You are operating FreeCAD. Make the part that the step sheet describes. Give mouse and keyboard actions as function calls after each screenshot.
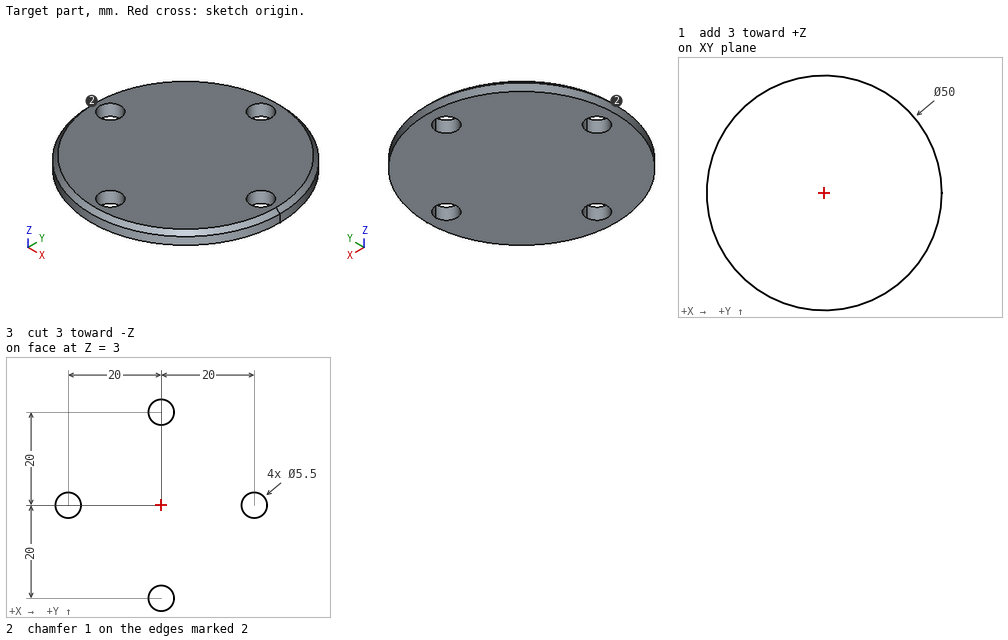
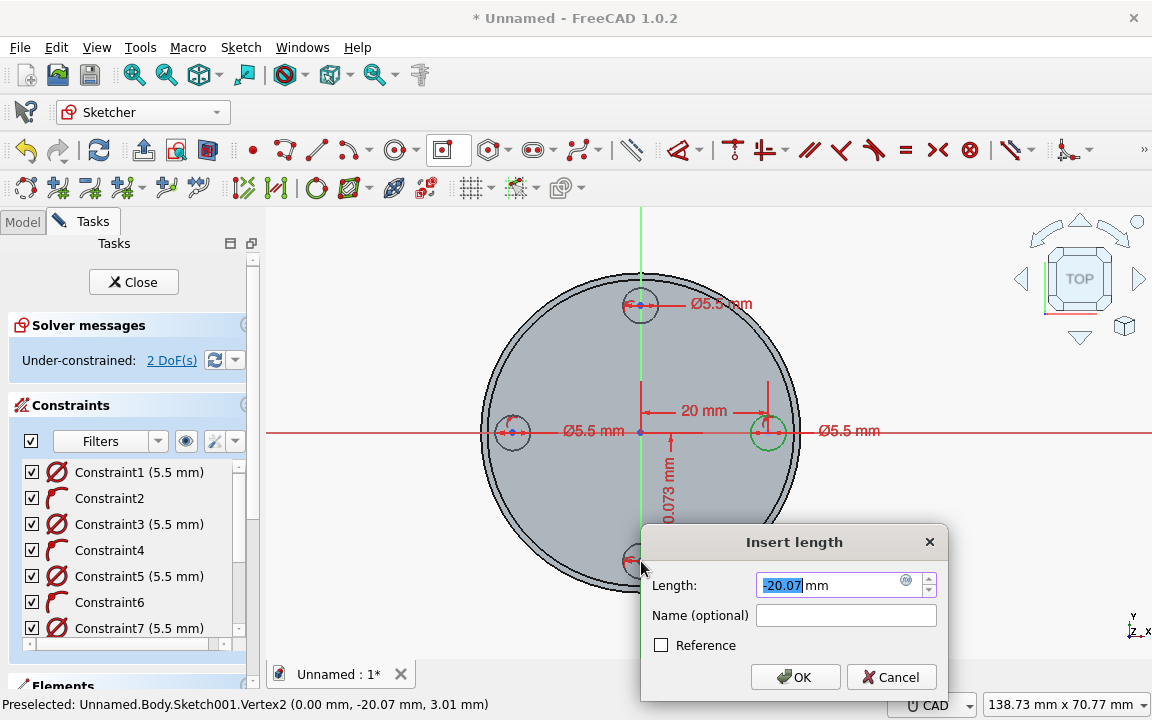
text(-20)
key(Return)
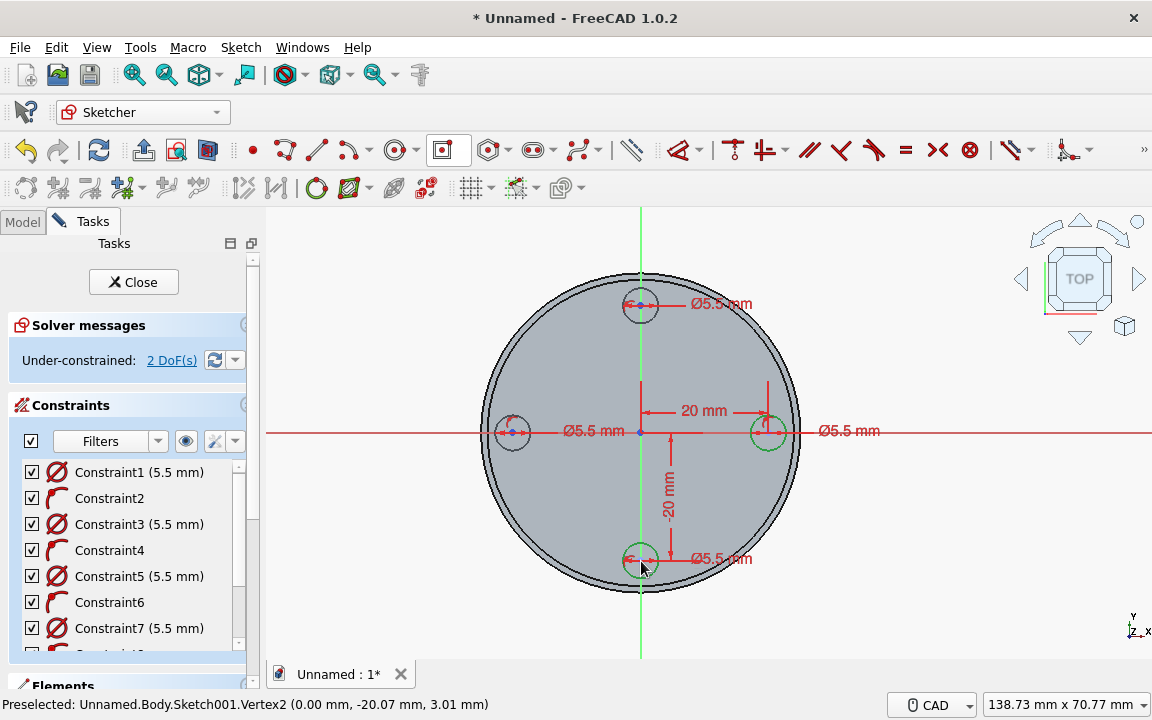
click(513, 433)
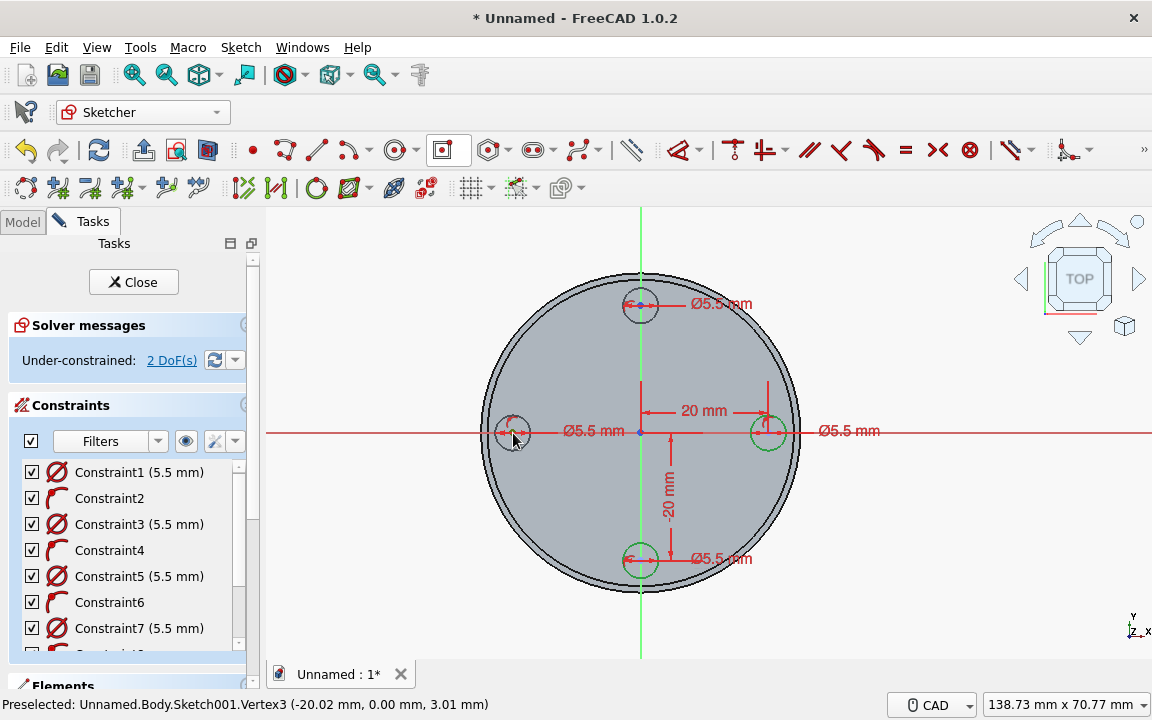
key(l)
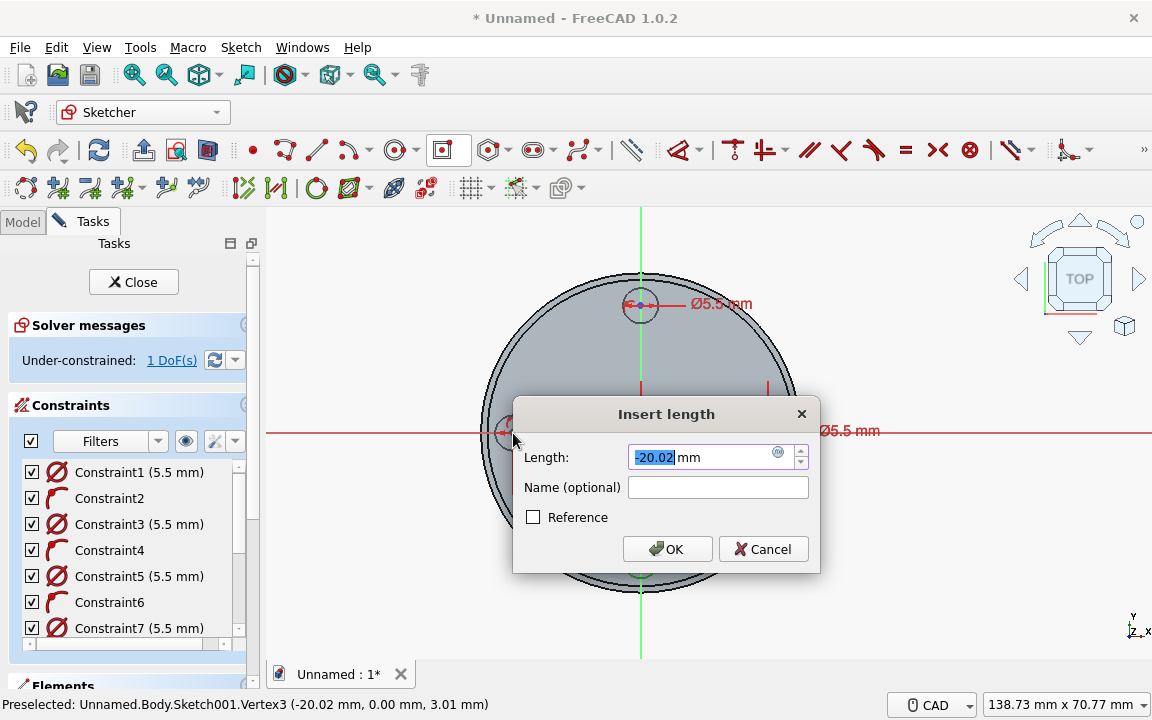
text(-20)
key(Return)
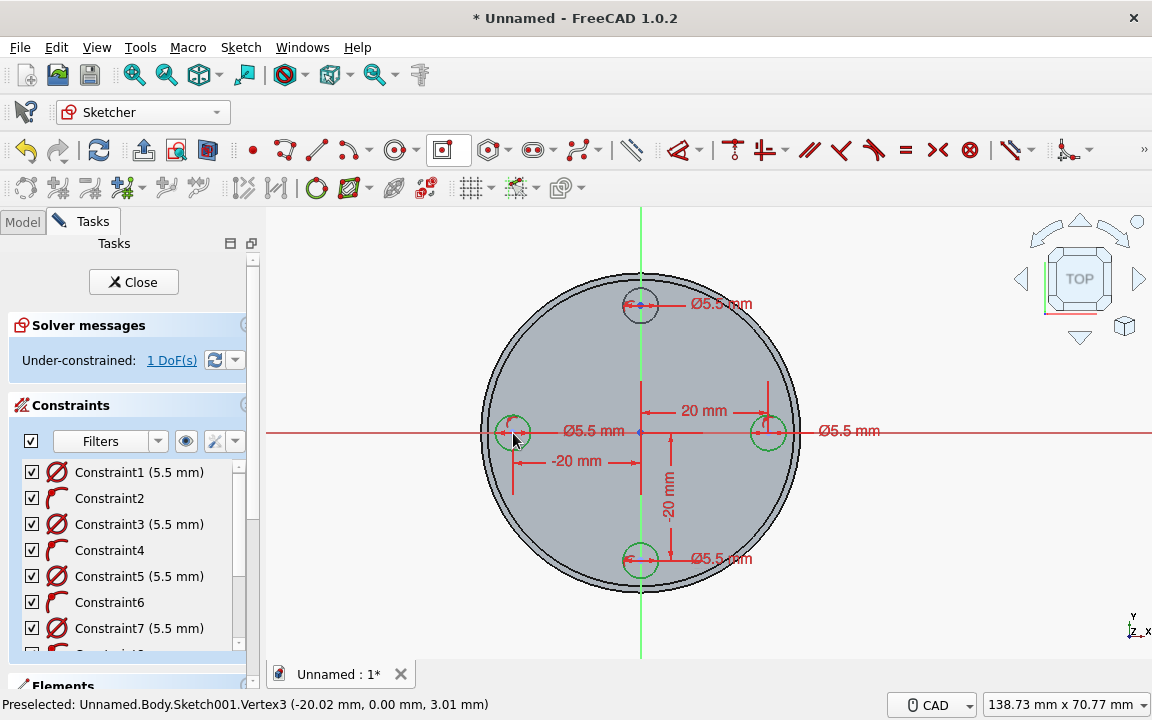
click(641, 306)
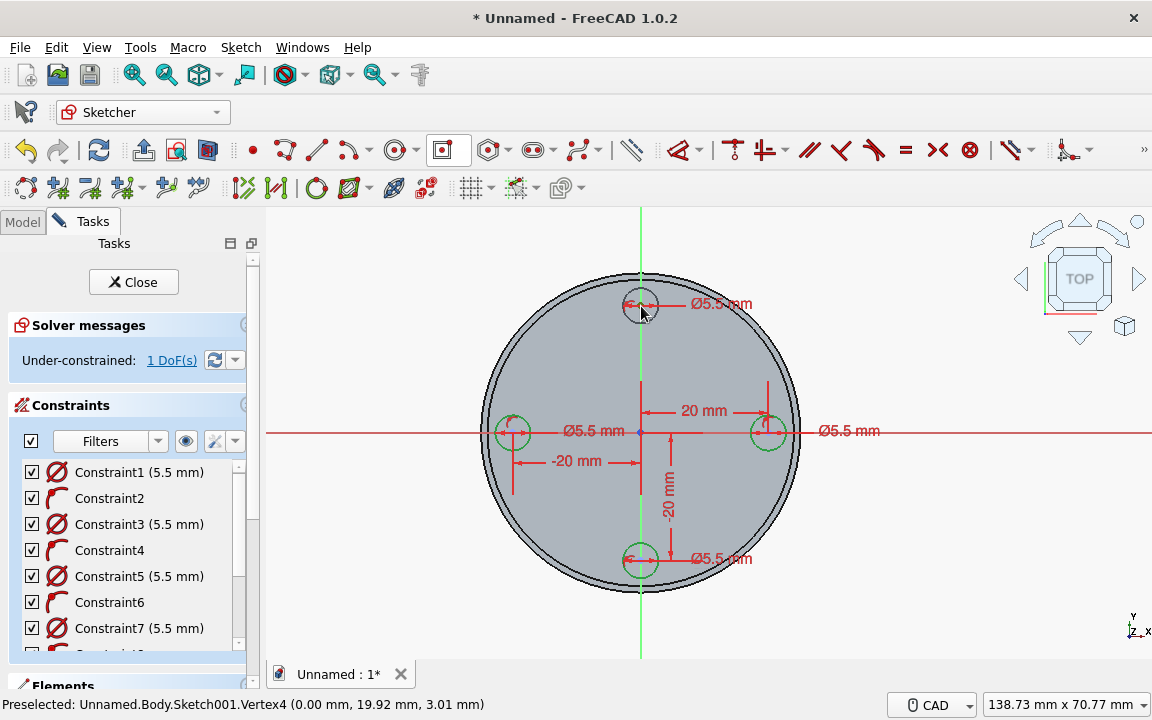
key(i)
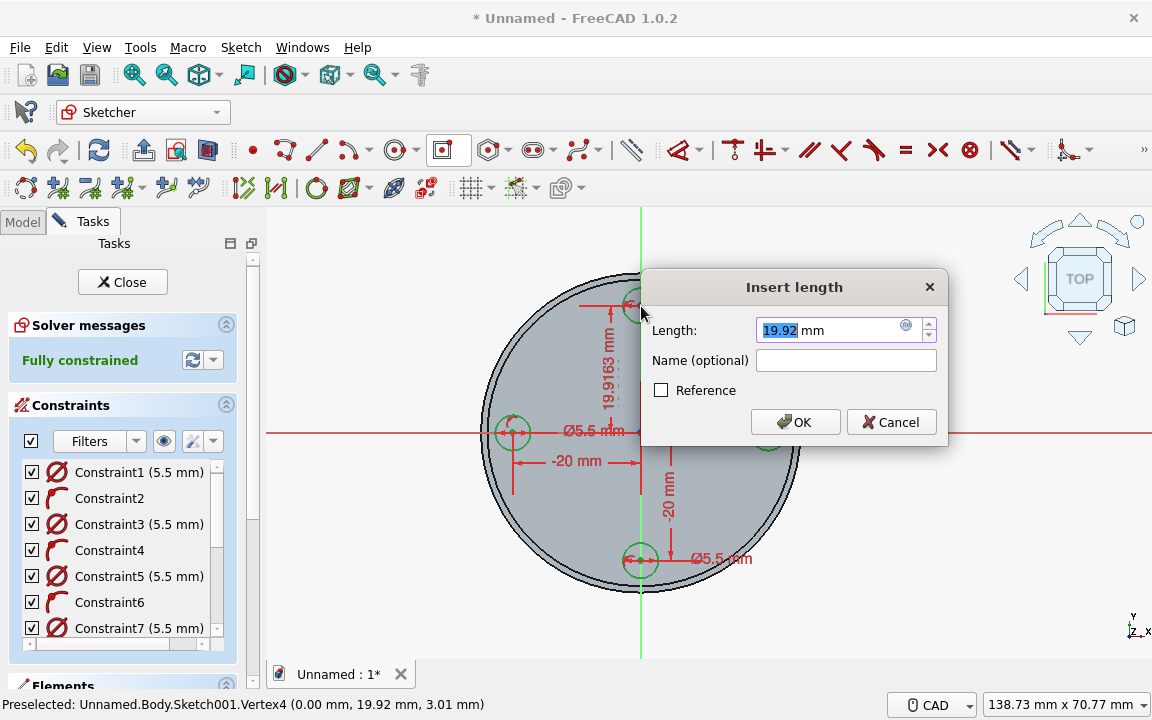
text(20)
key(Return)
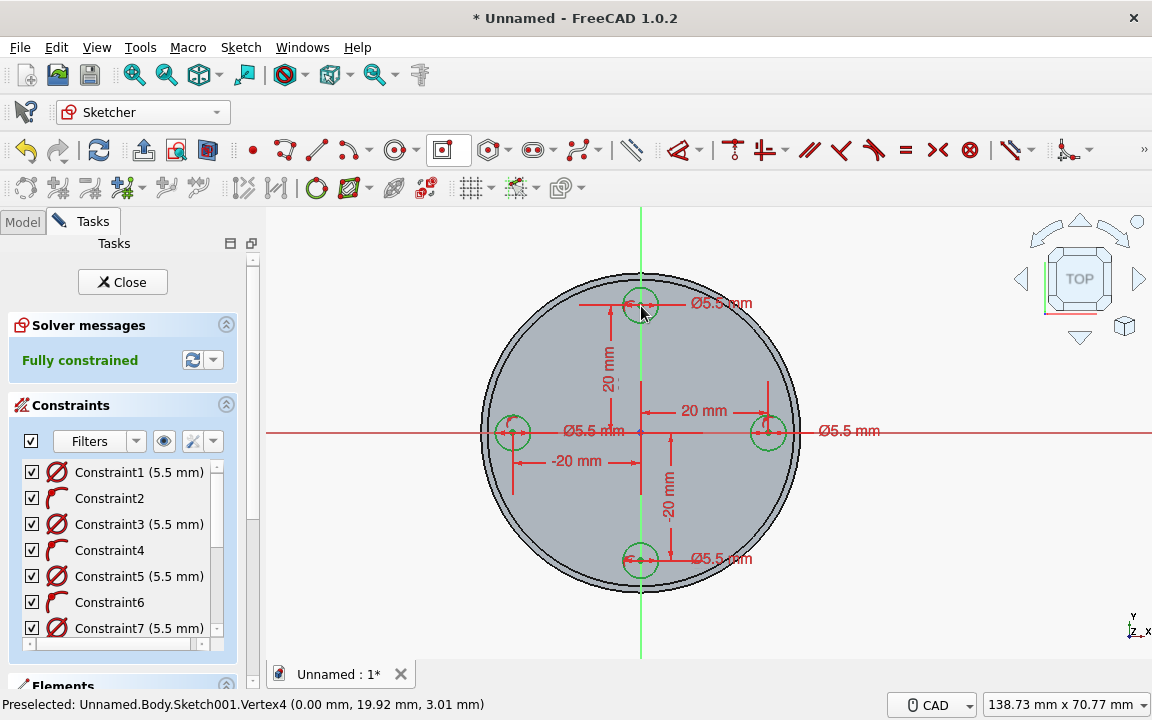
click(123, 282)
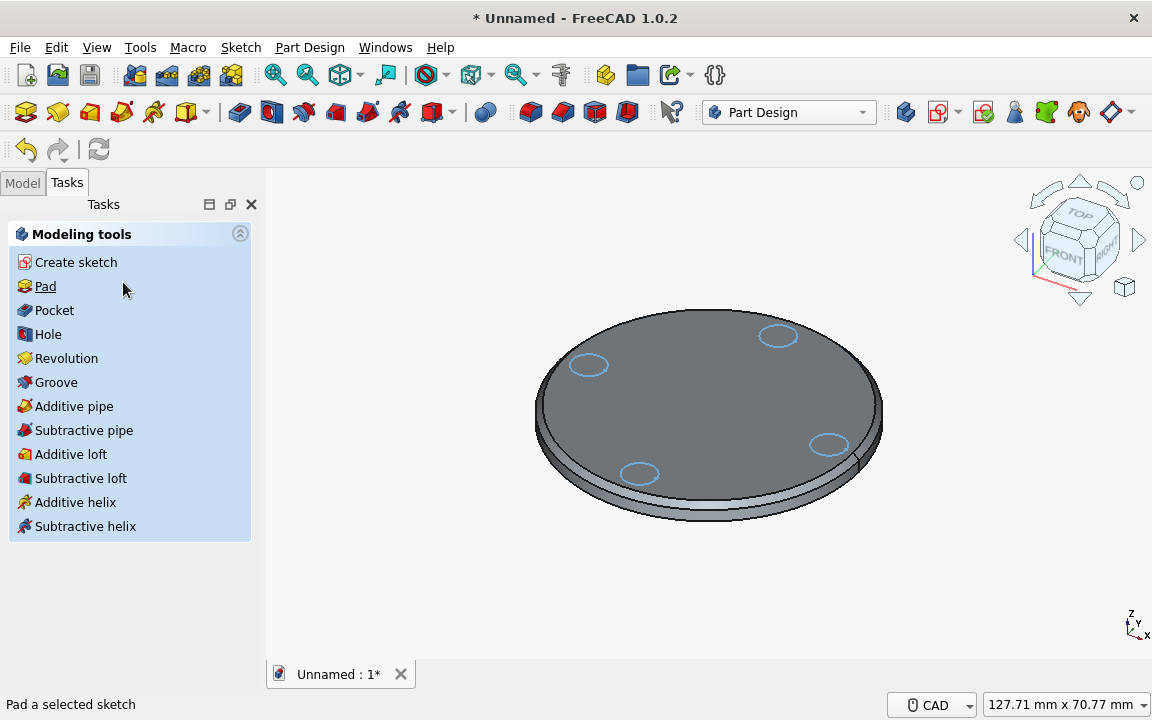
click(240, 112)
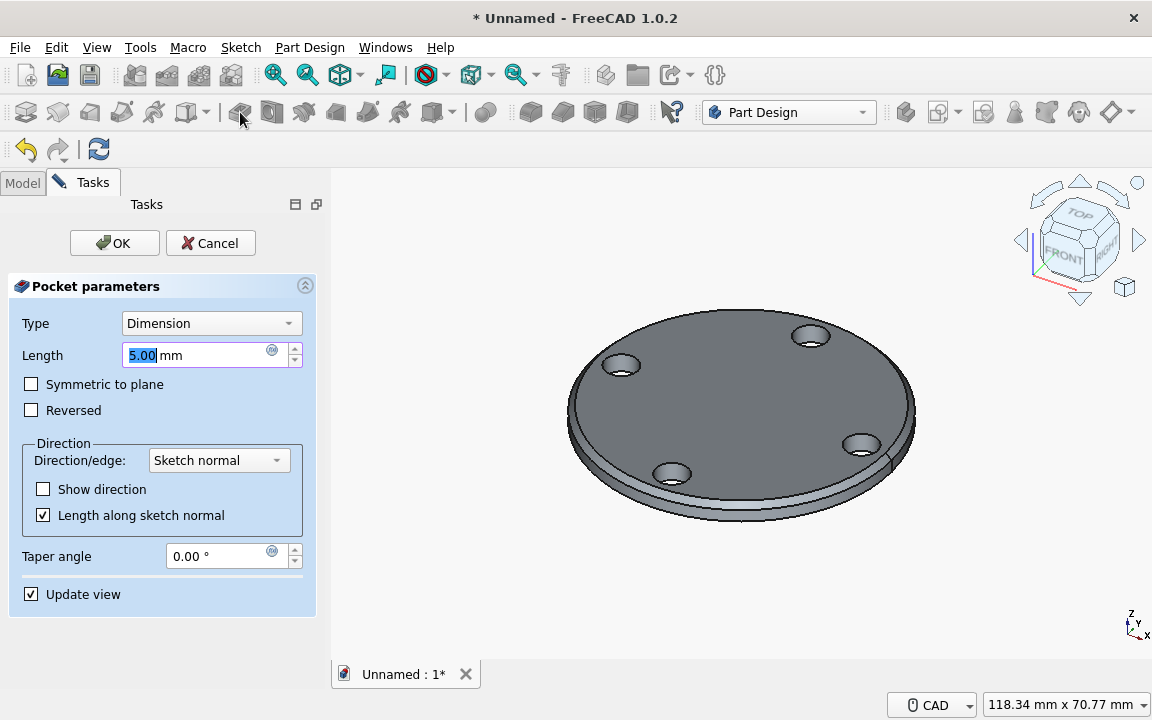
text(3)
key(Tab)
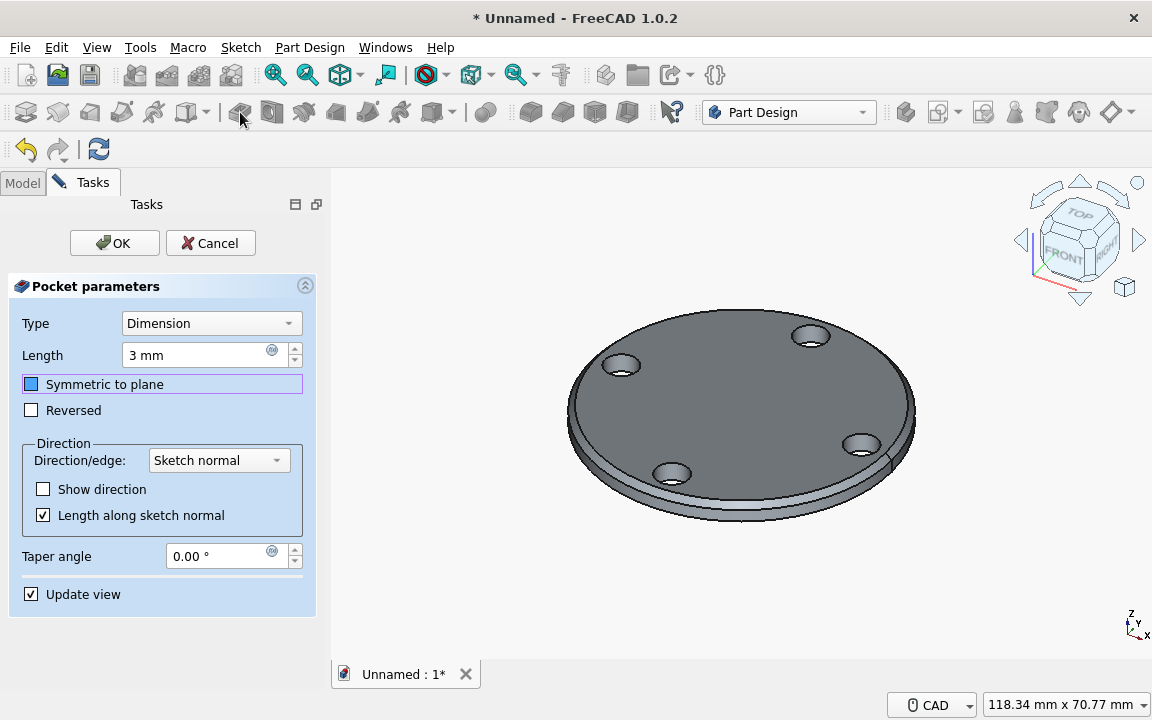
click(115, 243)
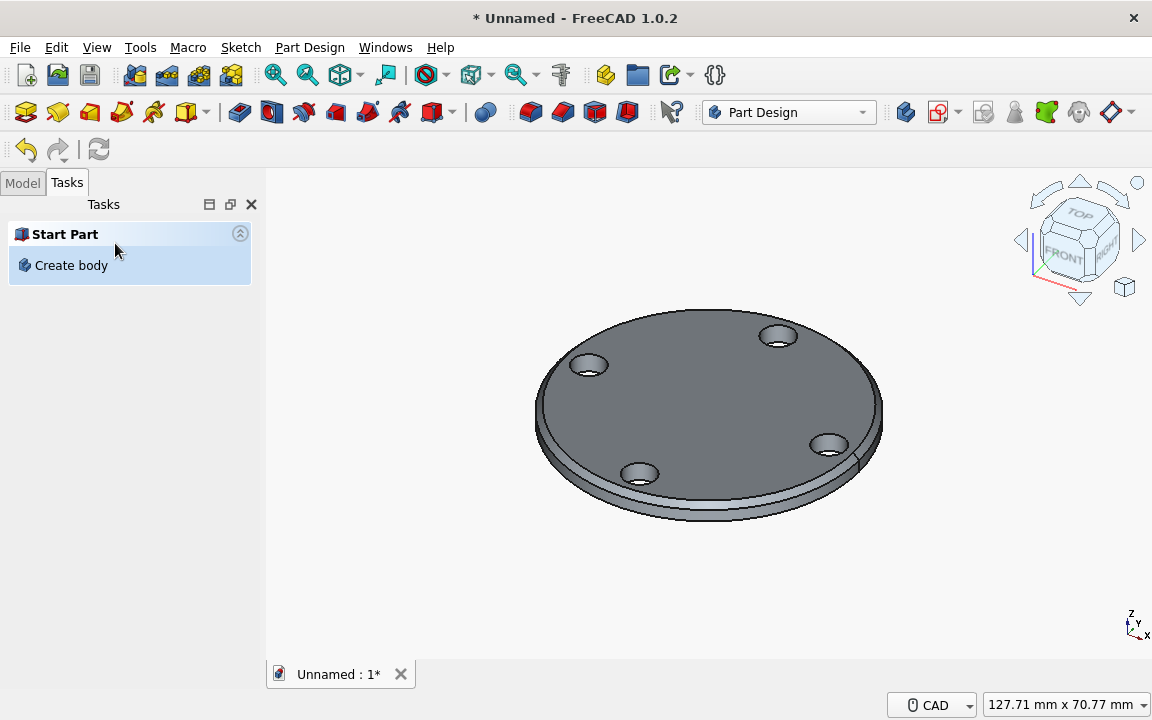
key(0)